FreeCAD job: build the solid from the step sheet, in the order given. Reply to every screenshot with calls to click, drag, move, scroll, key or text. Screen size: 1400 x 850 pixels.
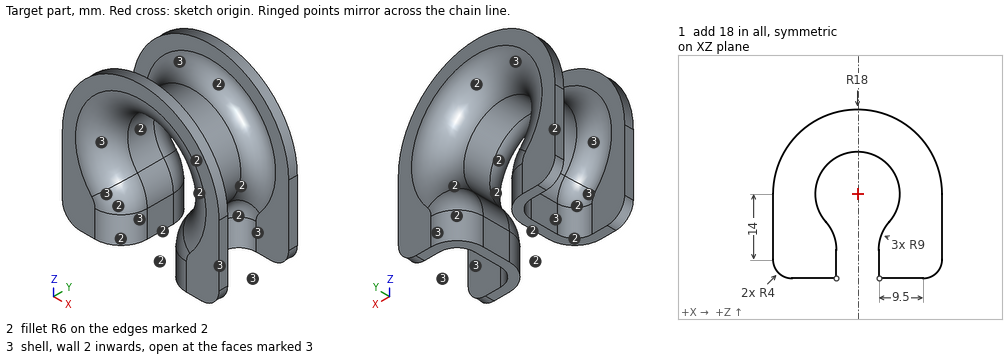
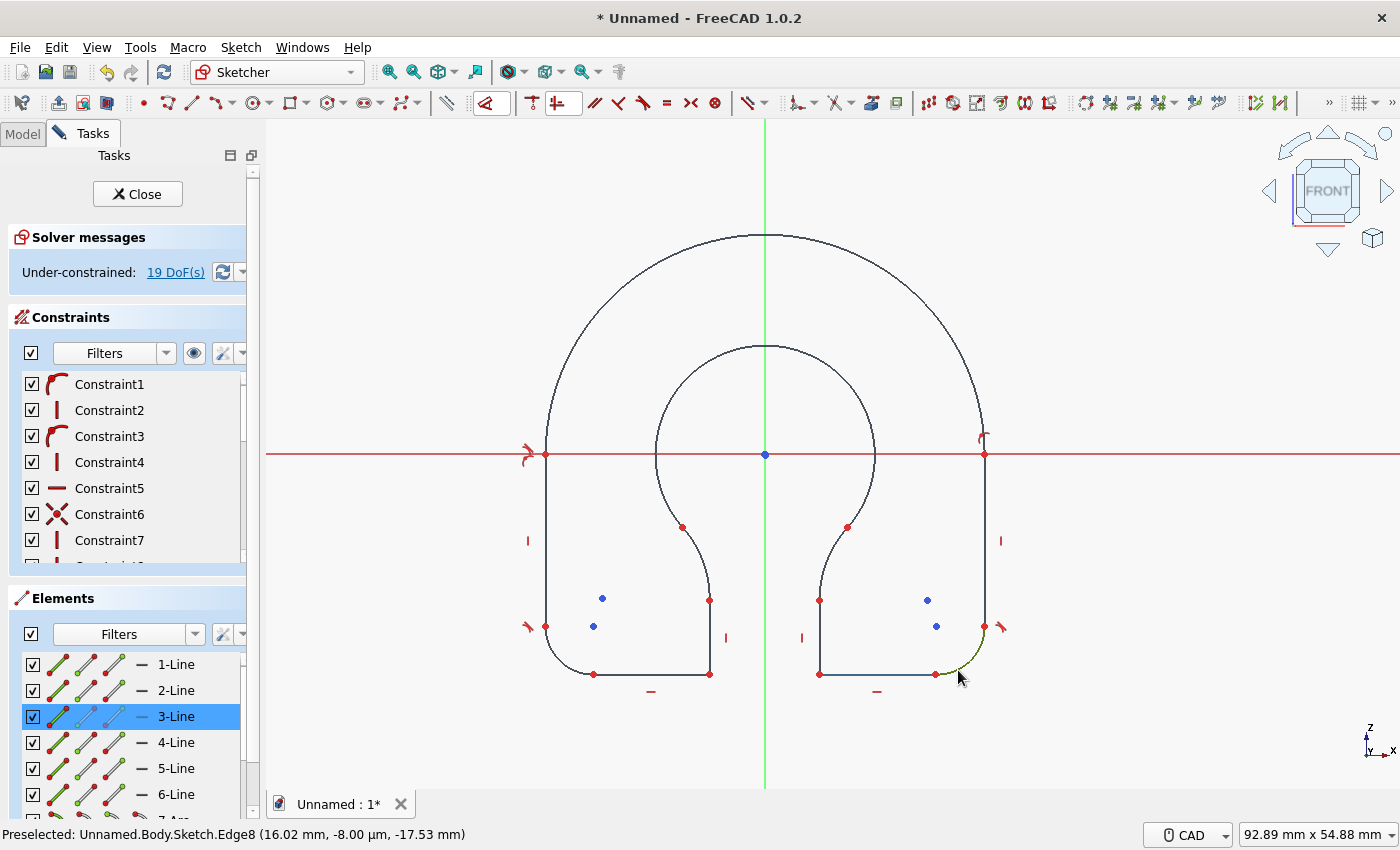
click(644, 104)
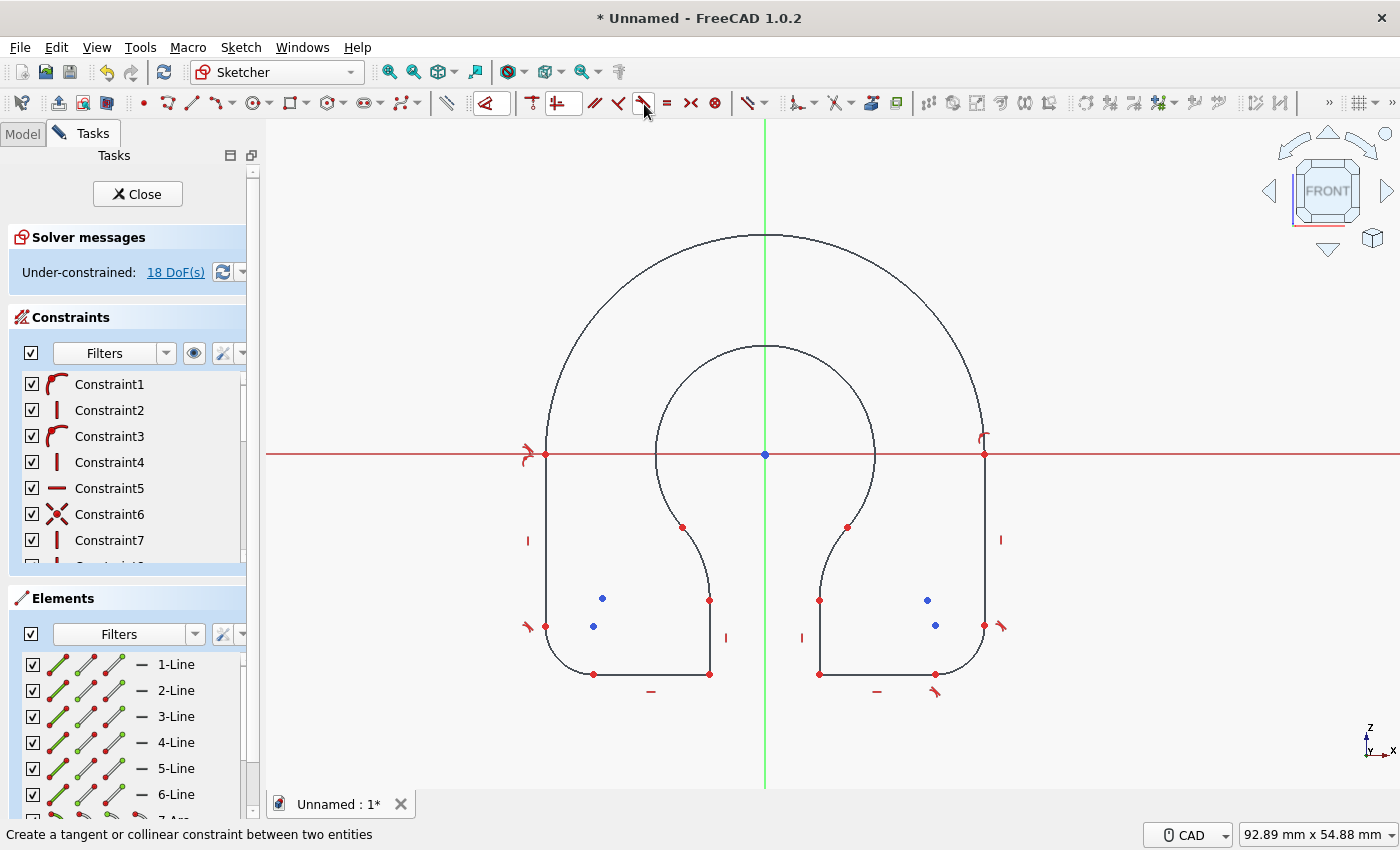
click(820, 652)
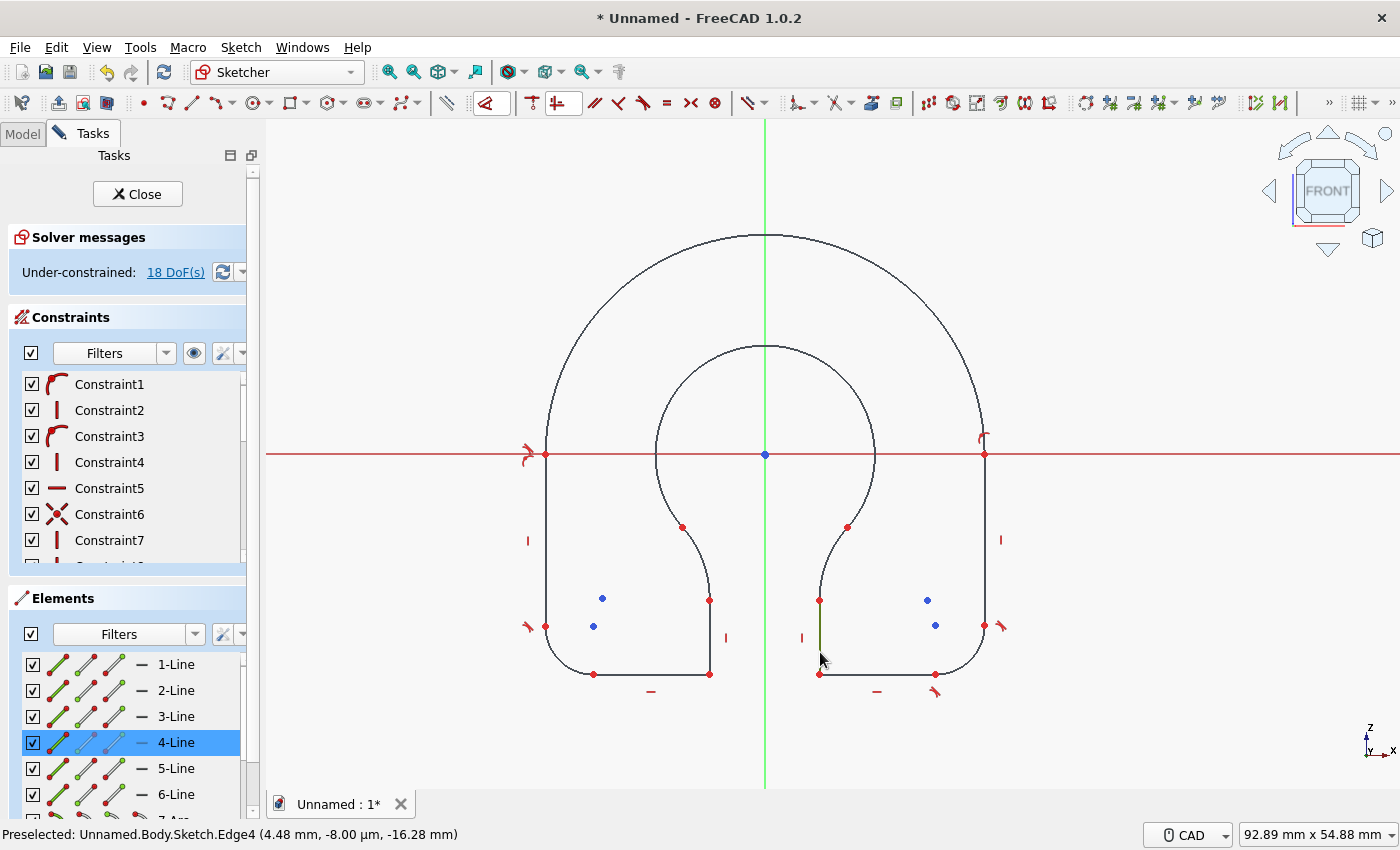
click(834, 547)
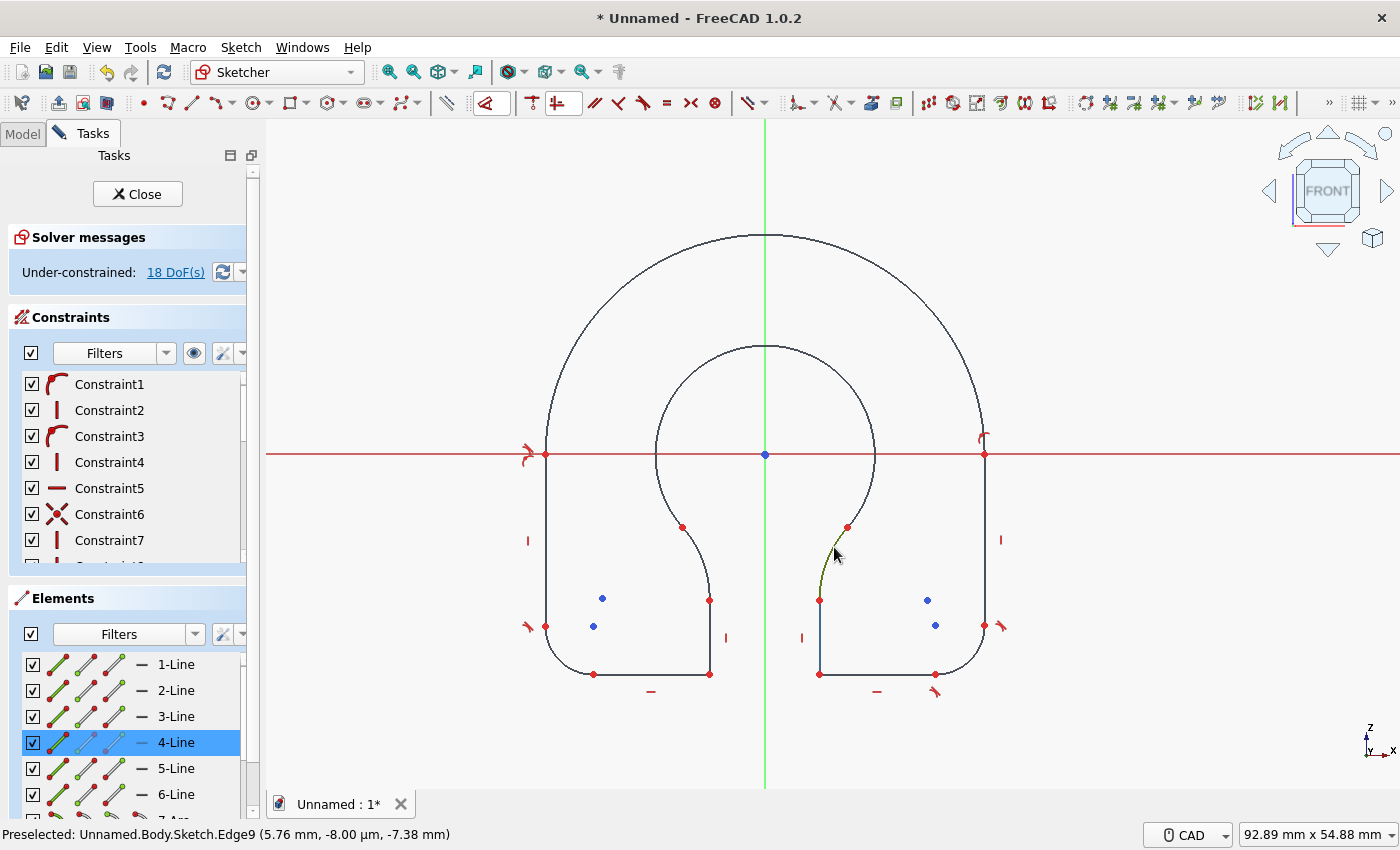
key(t)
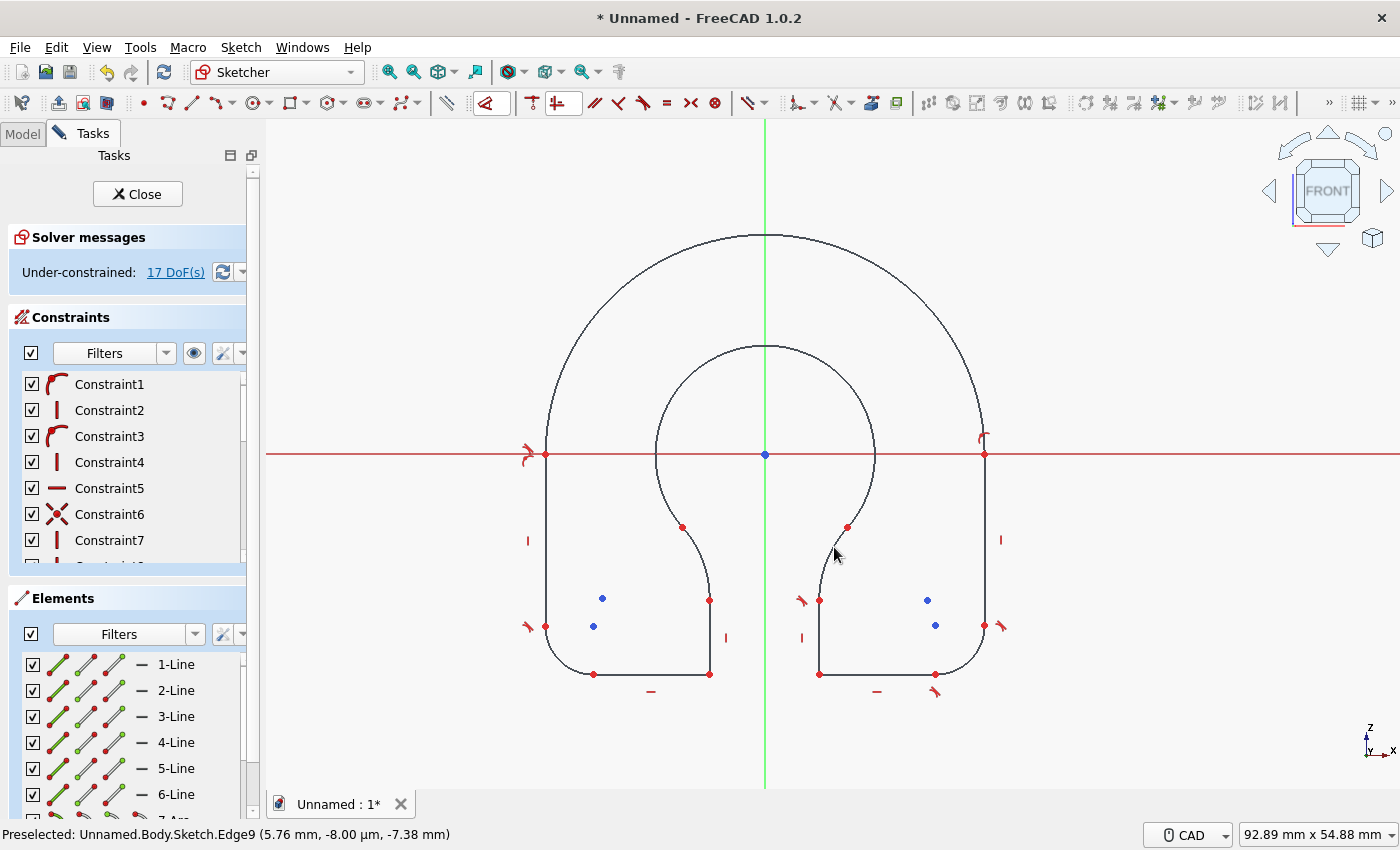
click(710, 623)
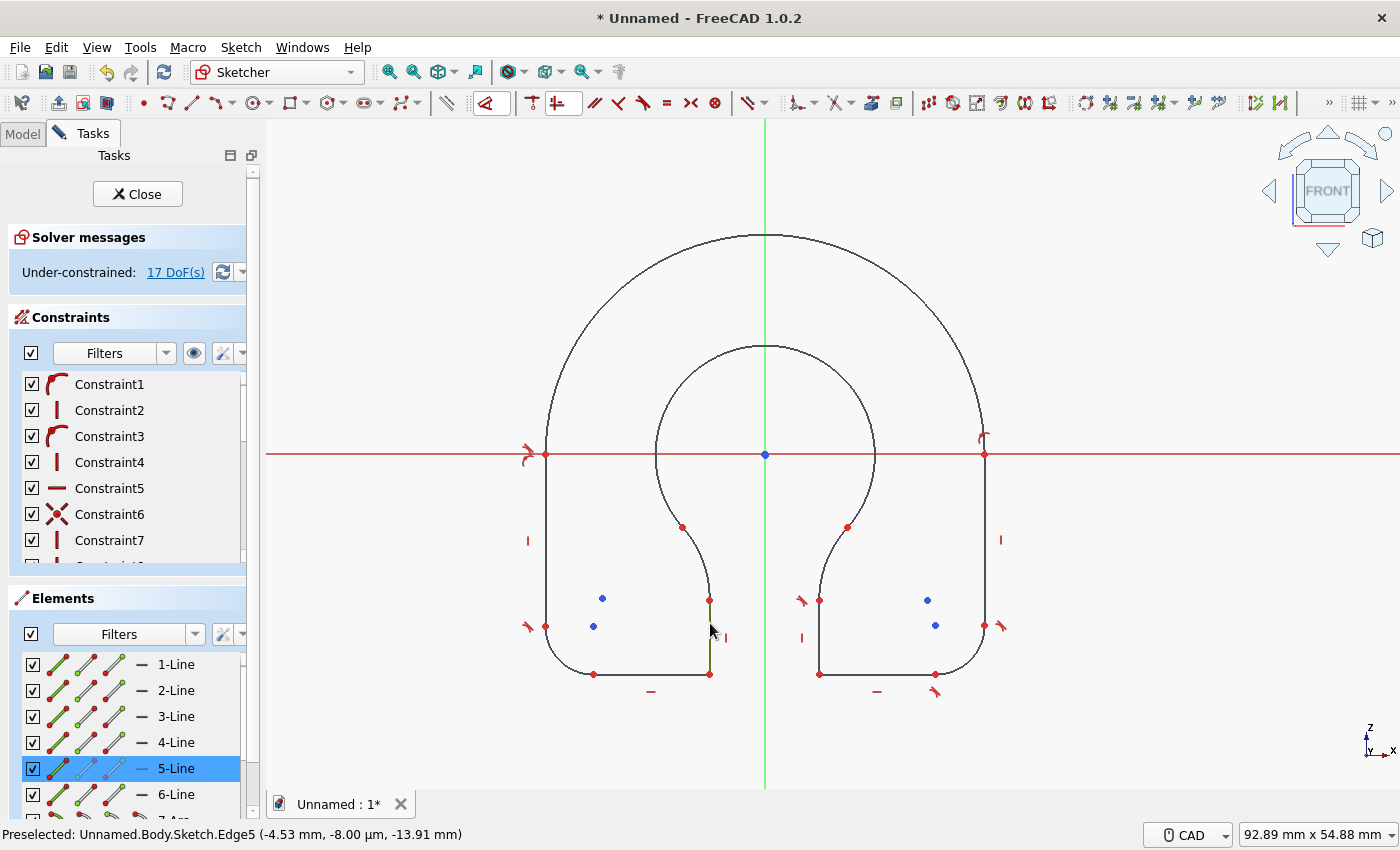
click(707, 577)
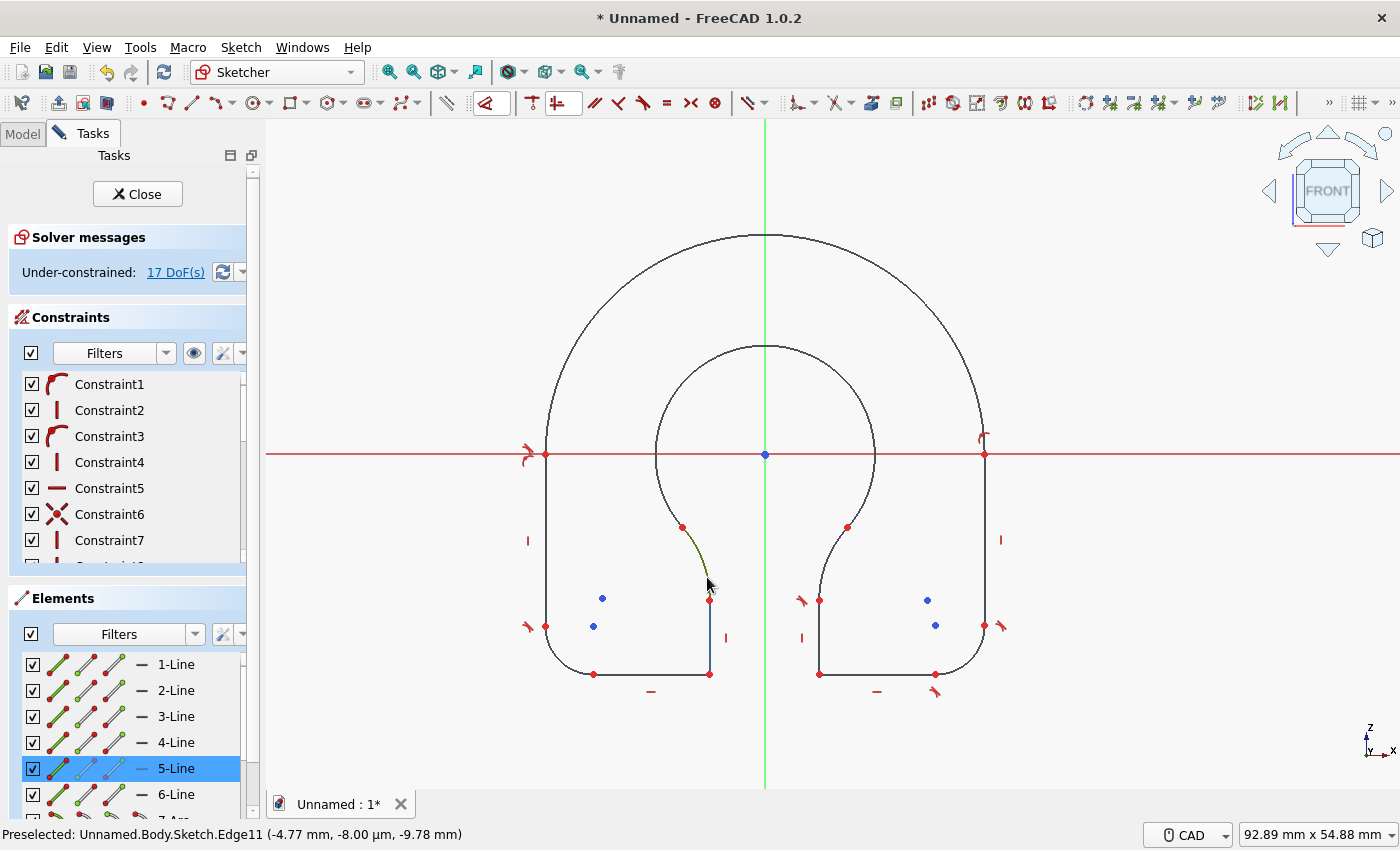
click(644, 104)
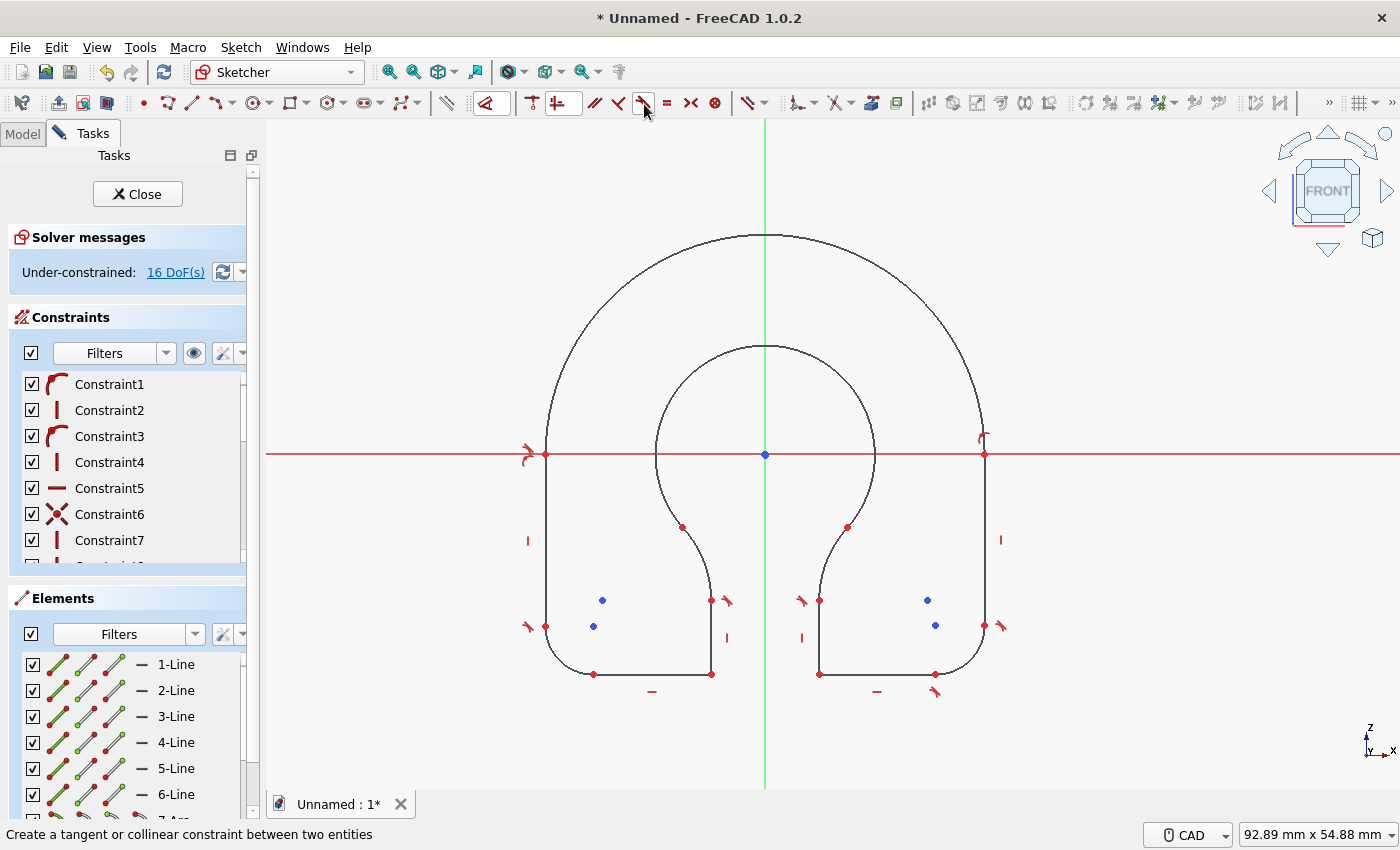
click(676, 675)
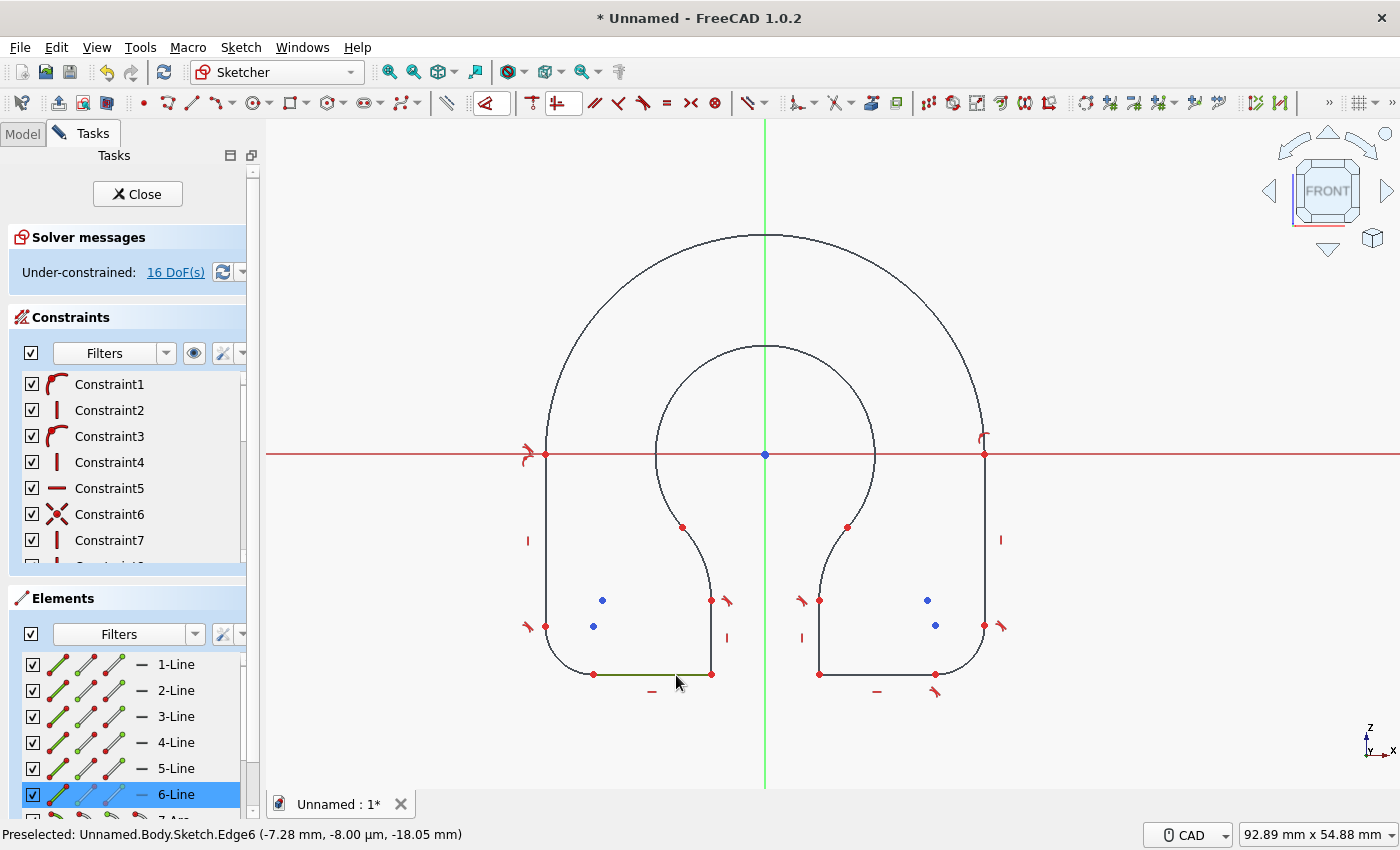
click(551, 648)